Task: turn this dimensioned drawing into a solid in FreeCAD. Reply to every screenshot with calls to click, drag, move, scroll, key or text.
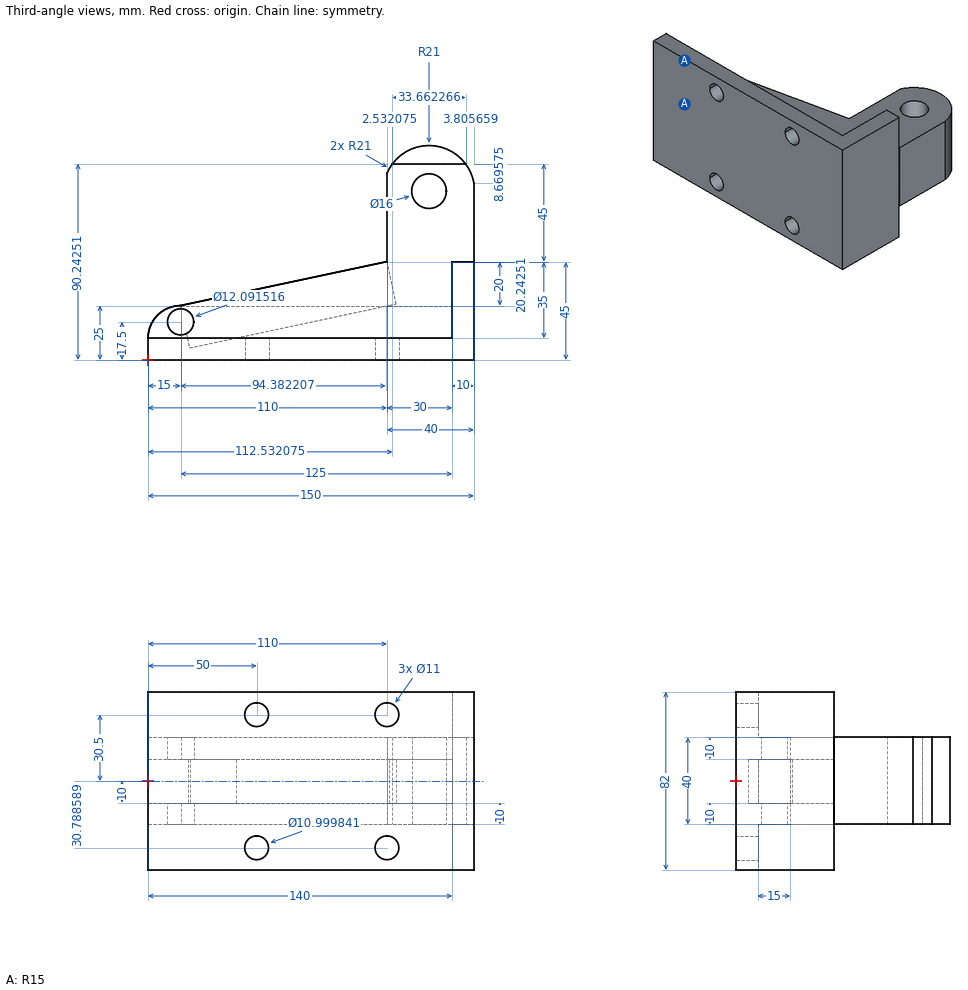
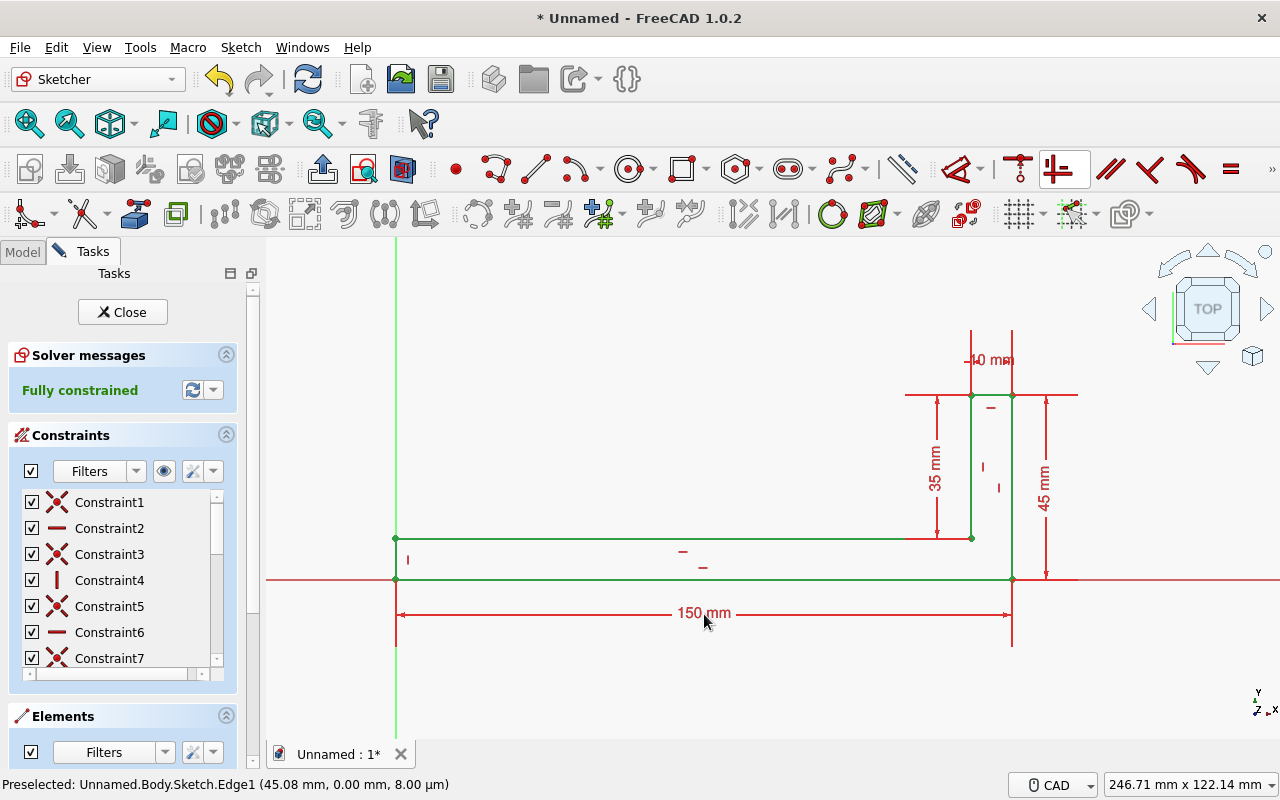
click(123, 312)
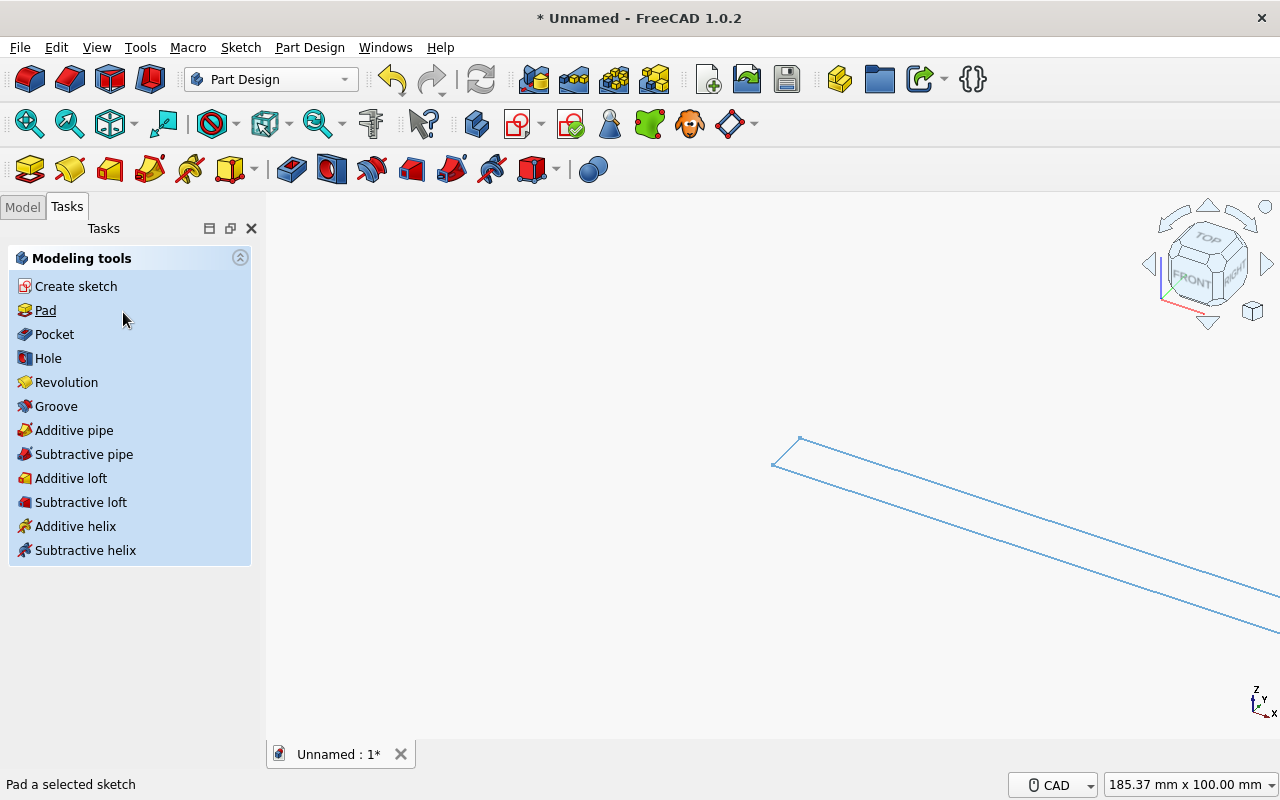
click(30, 170)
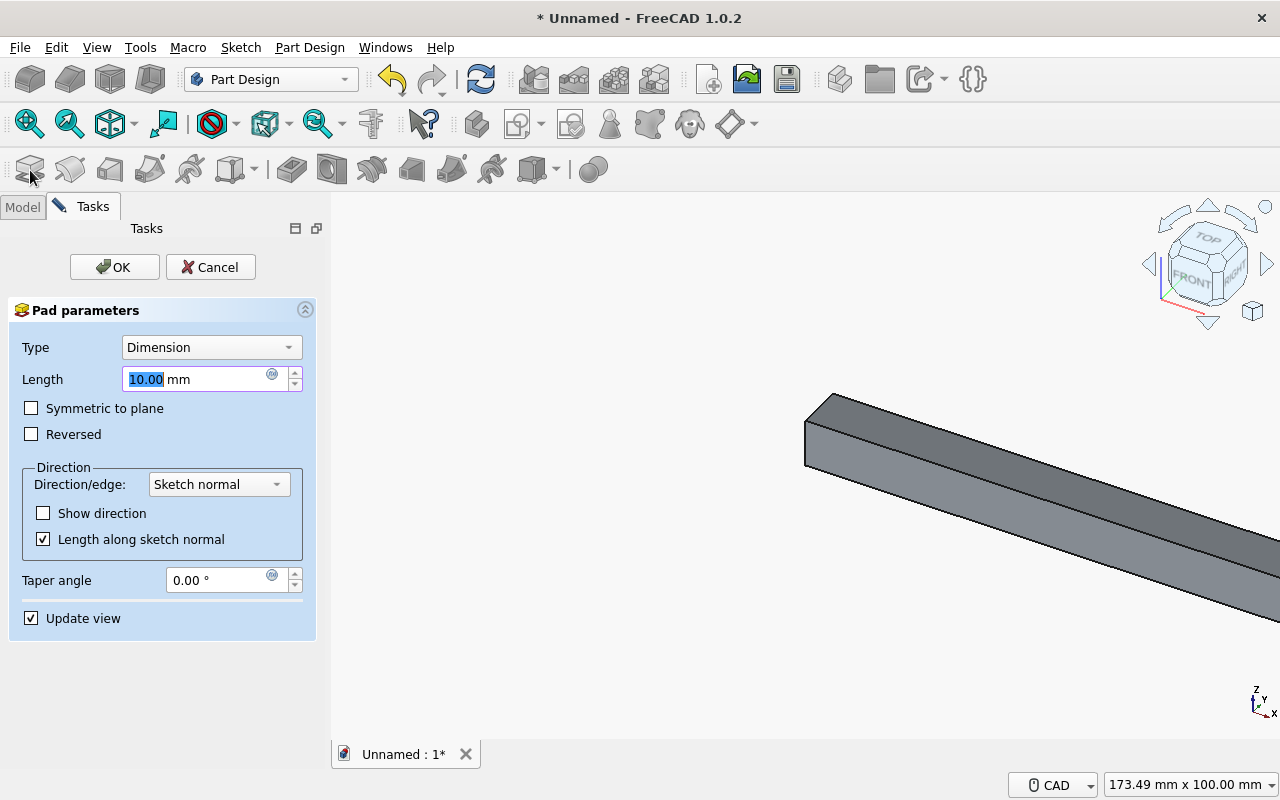
text(82)
key(Tab)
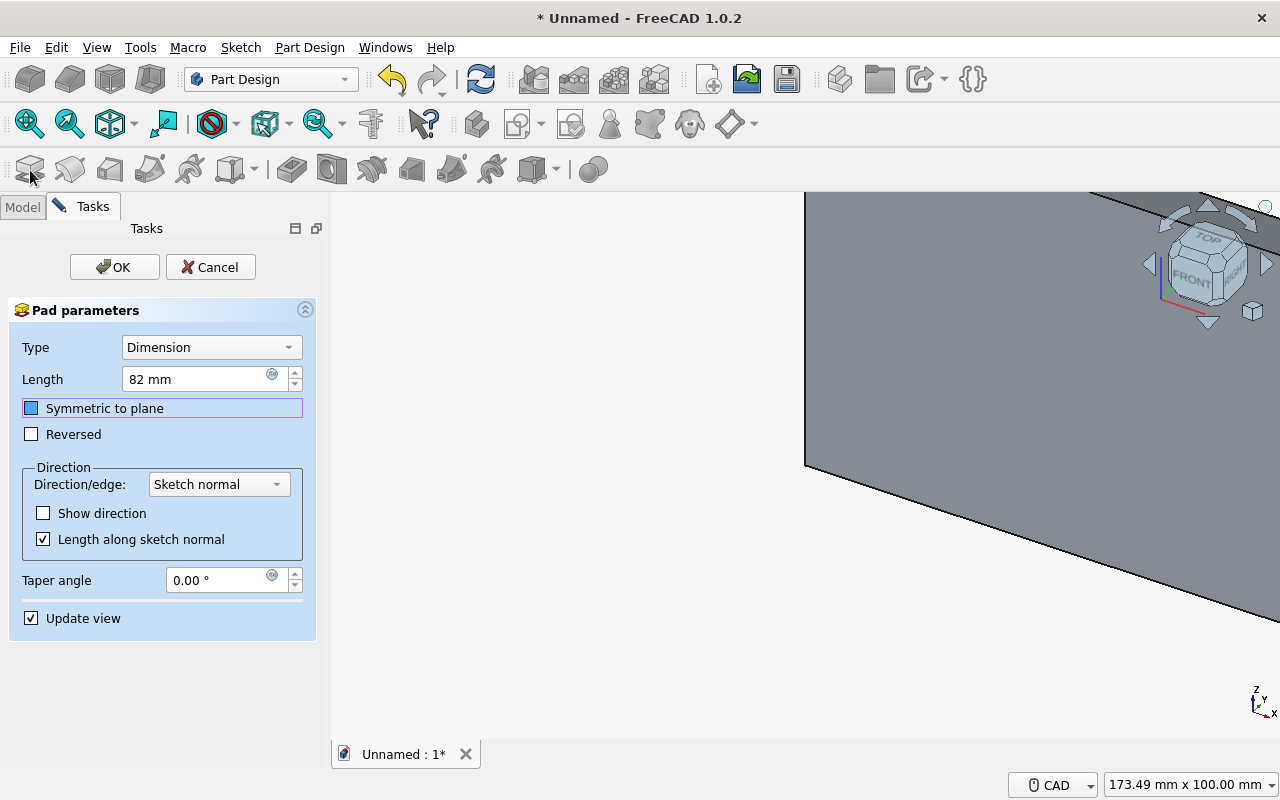
click(30, 408)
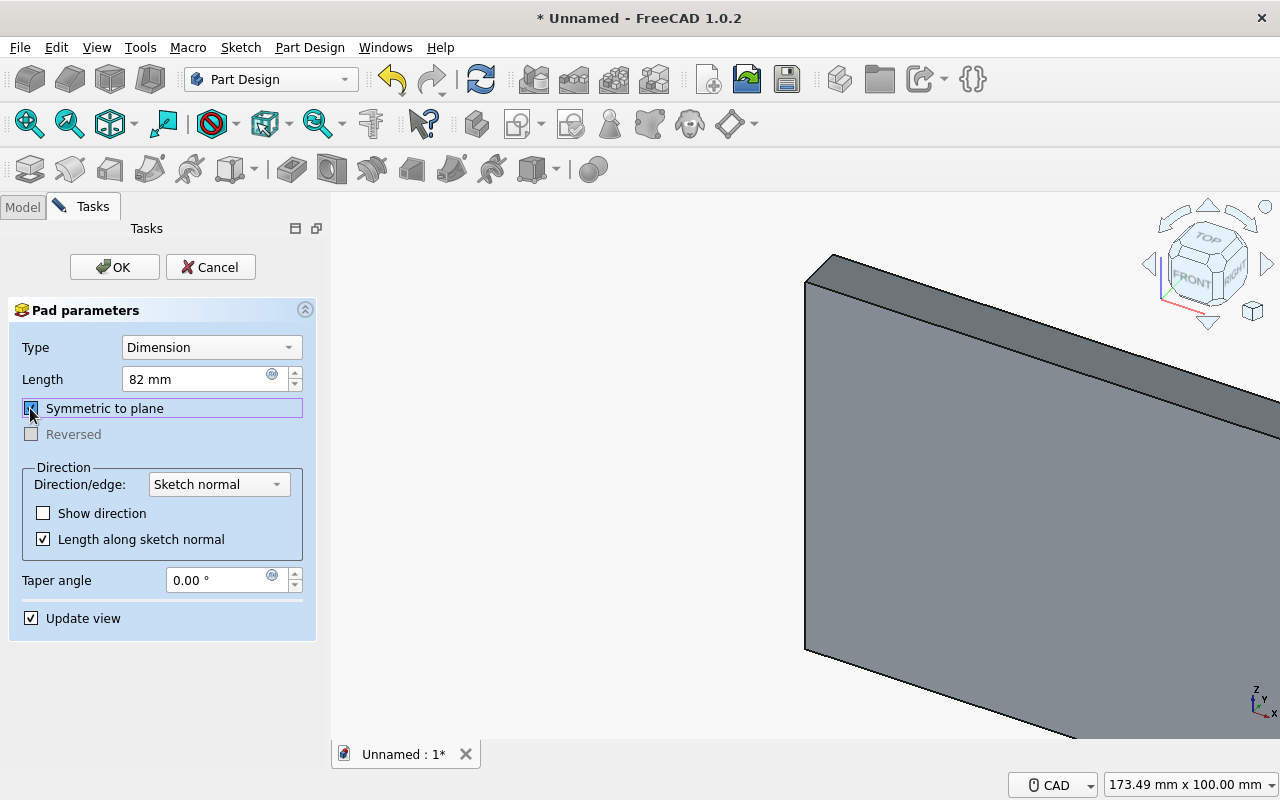
click(115, 267)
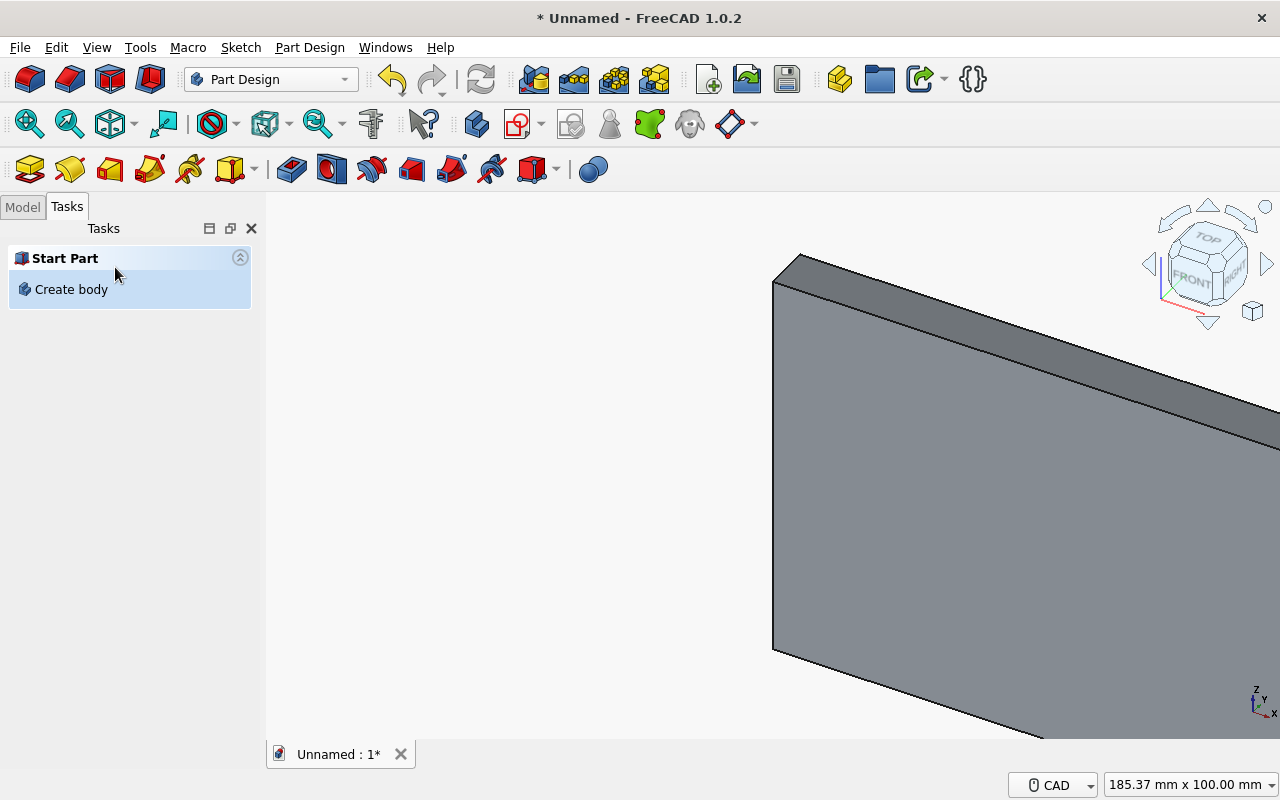
click(30, 124)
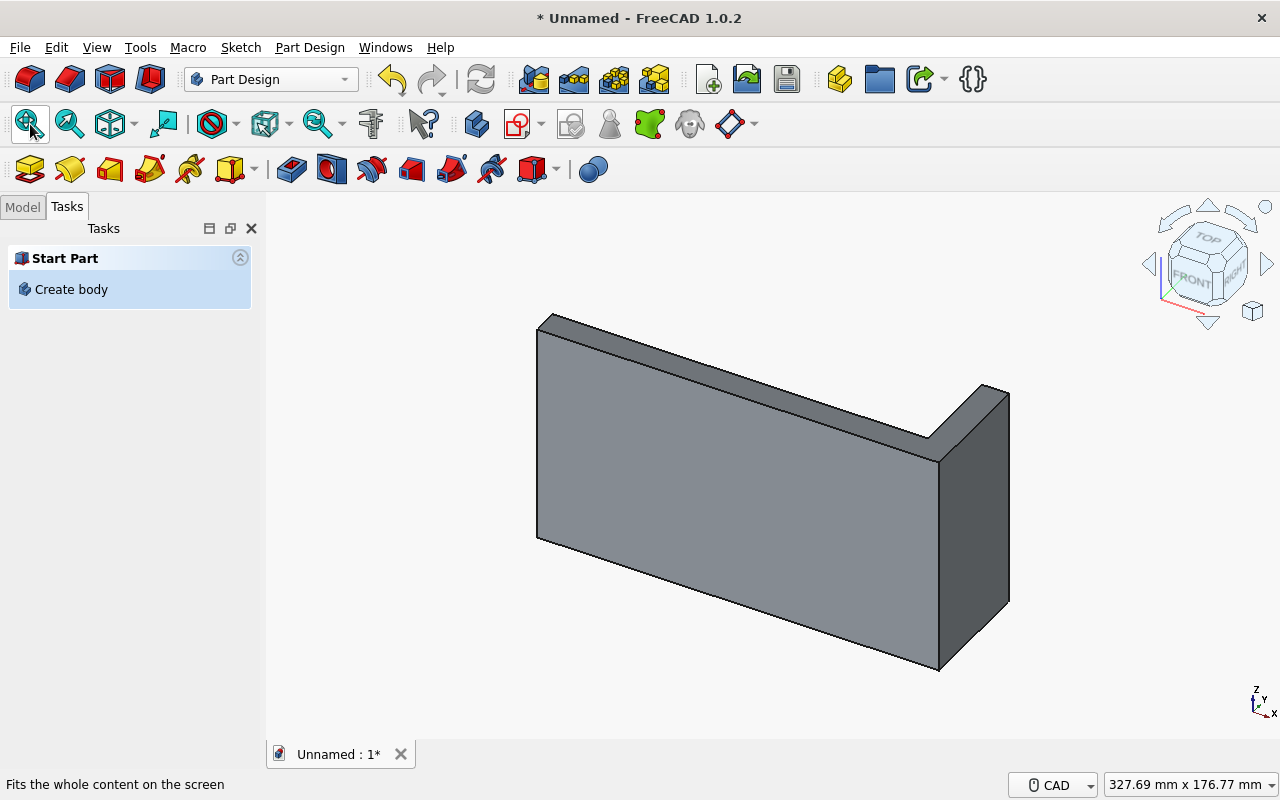
key(4)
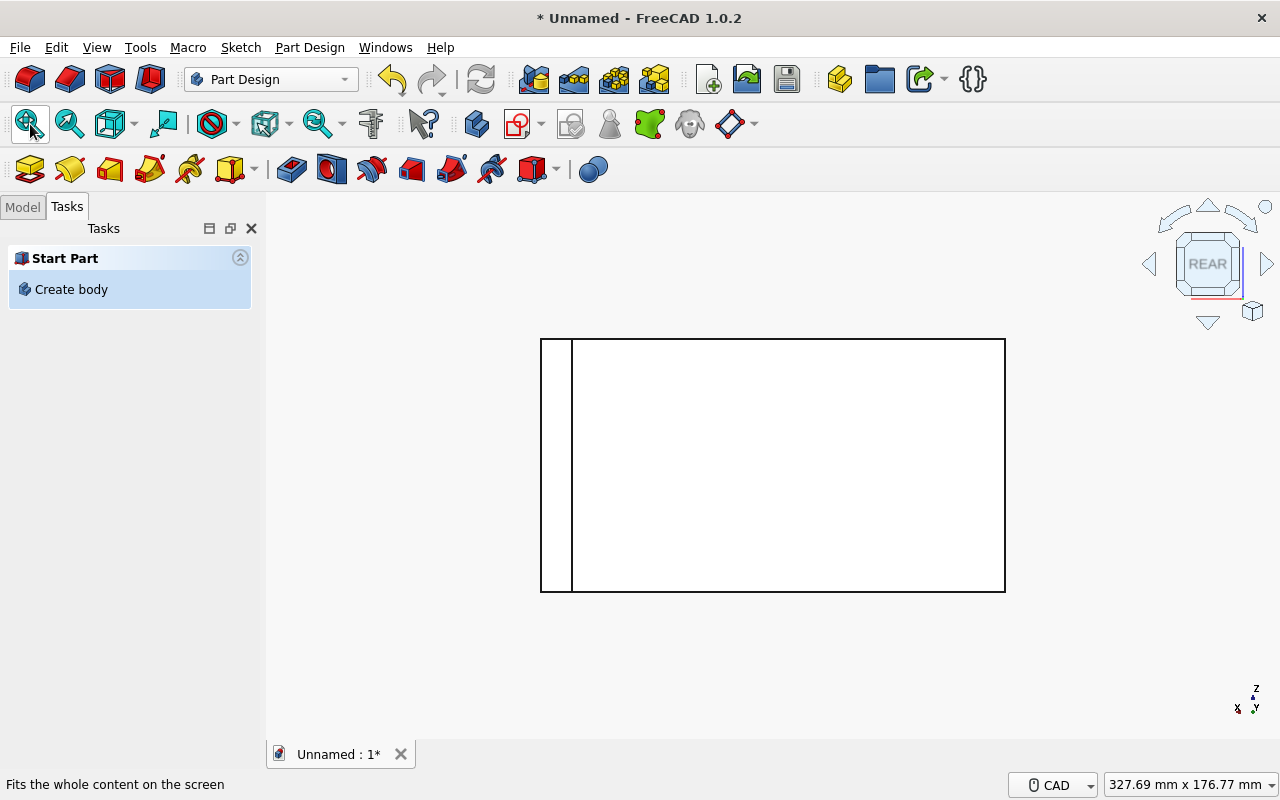
click(727, 465)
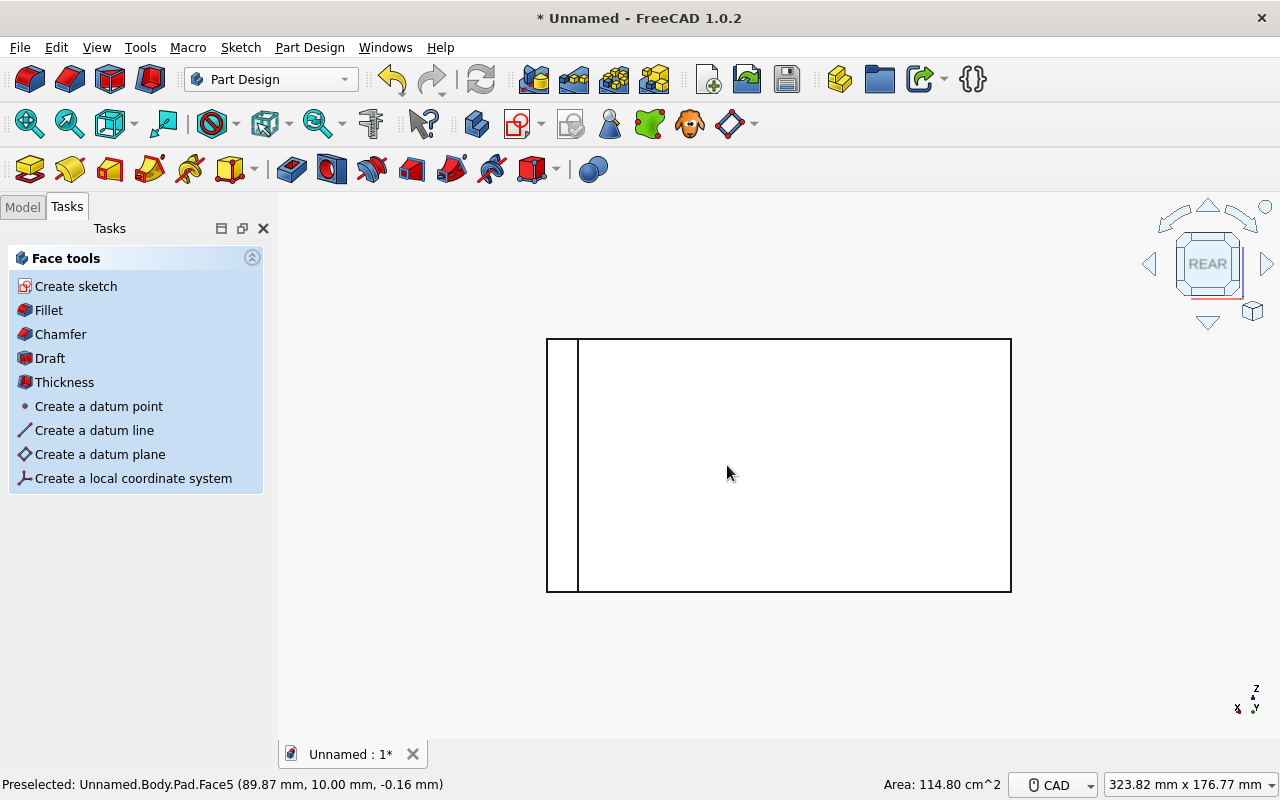
click(518, 124)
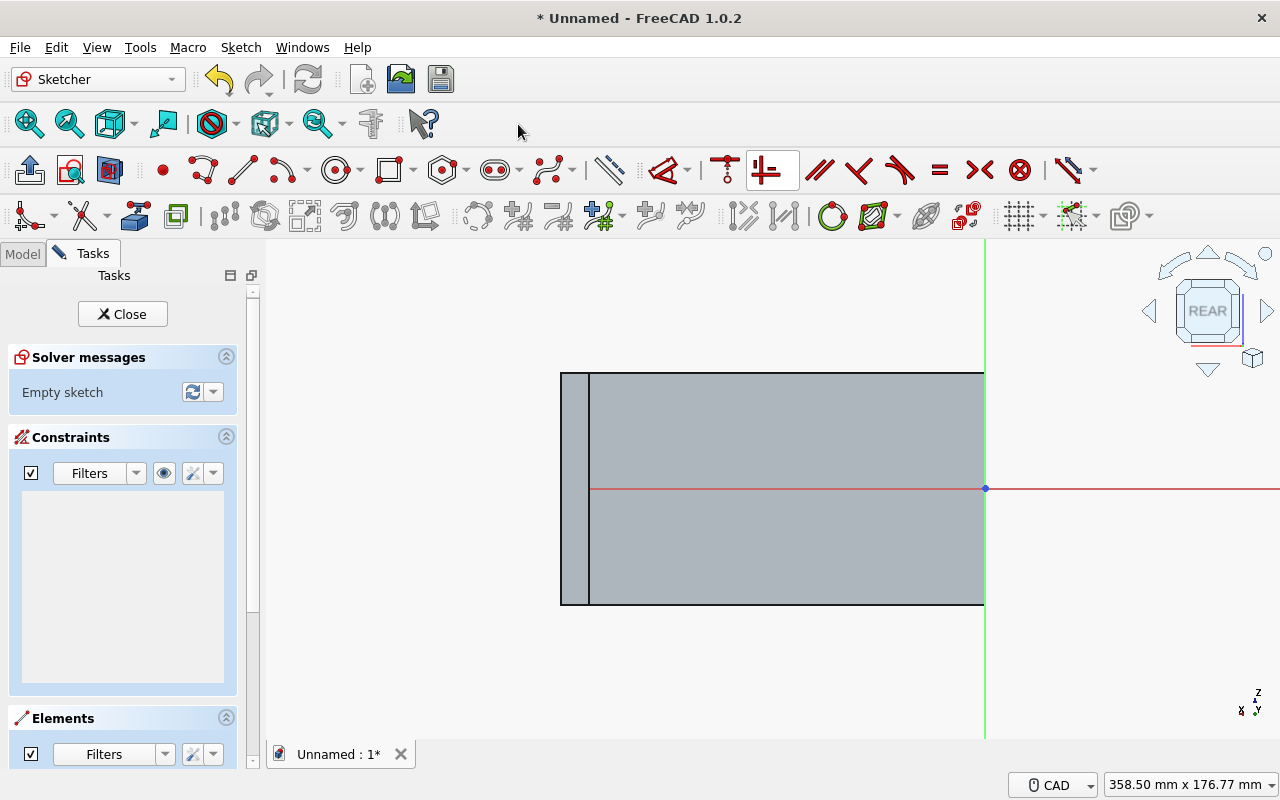
key(q)
key(s)